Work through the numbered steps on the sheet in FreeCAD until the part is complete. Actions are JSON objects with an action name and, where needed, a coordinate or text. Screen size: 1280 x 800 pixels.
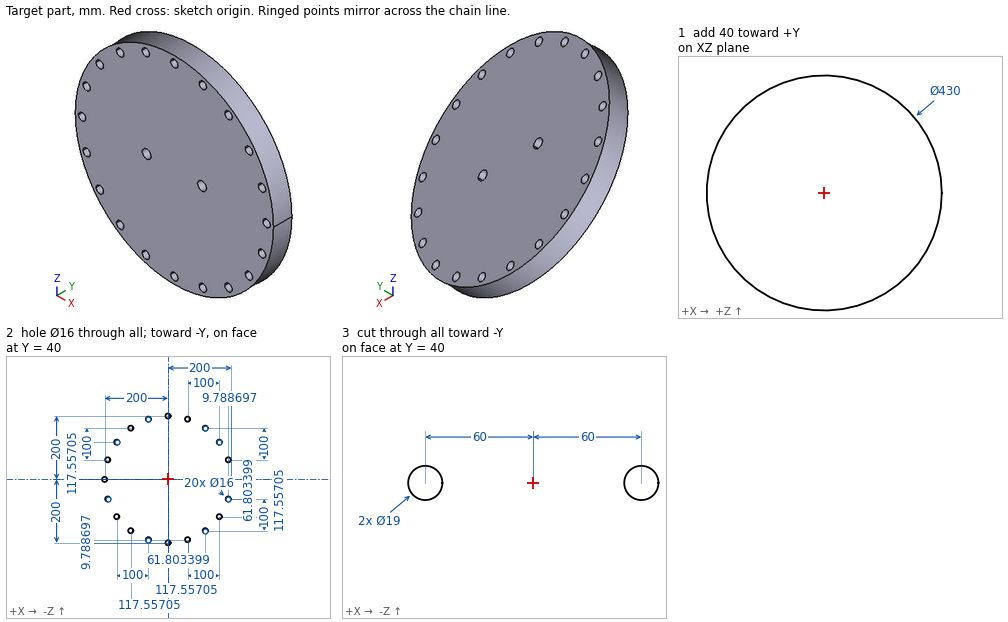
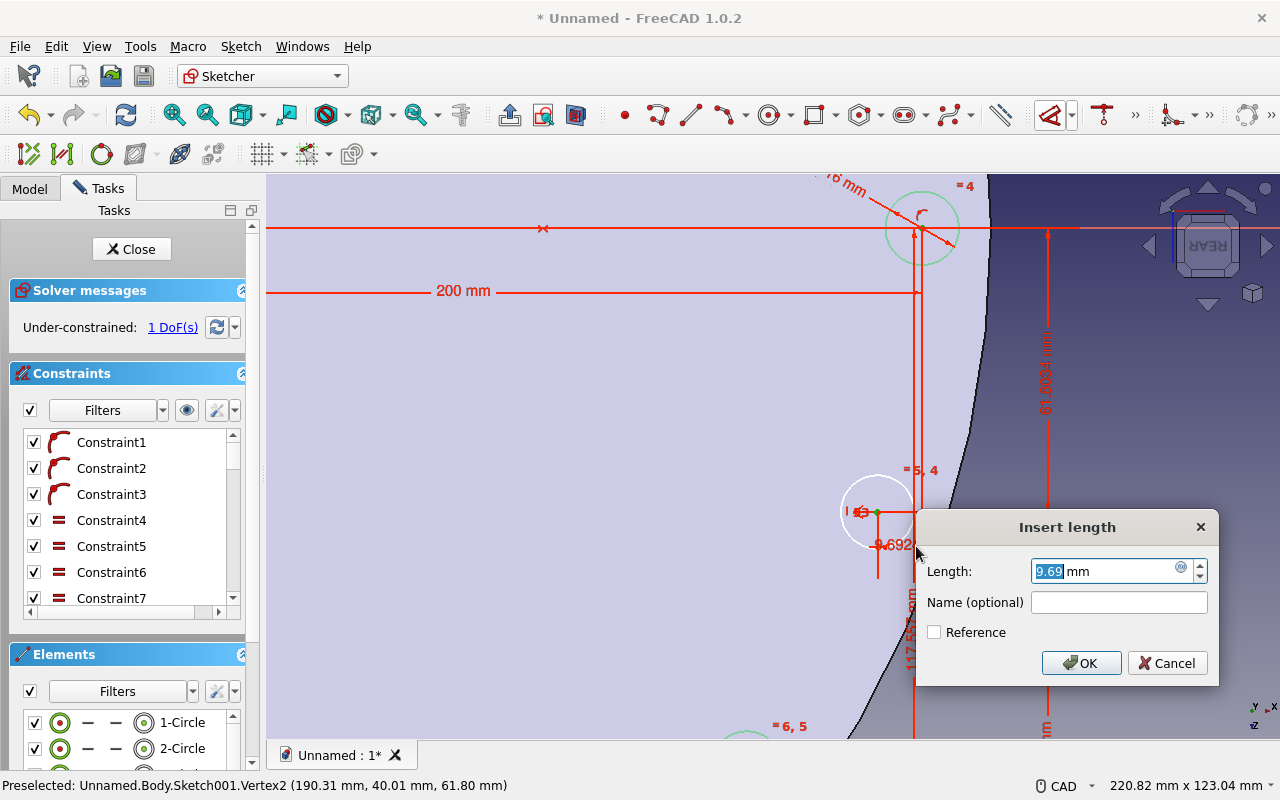
{"action": "type", "text": "9.788697"}
{"action": "key", "text": "Return"}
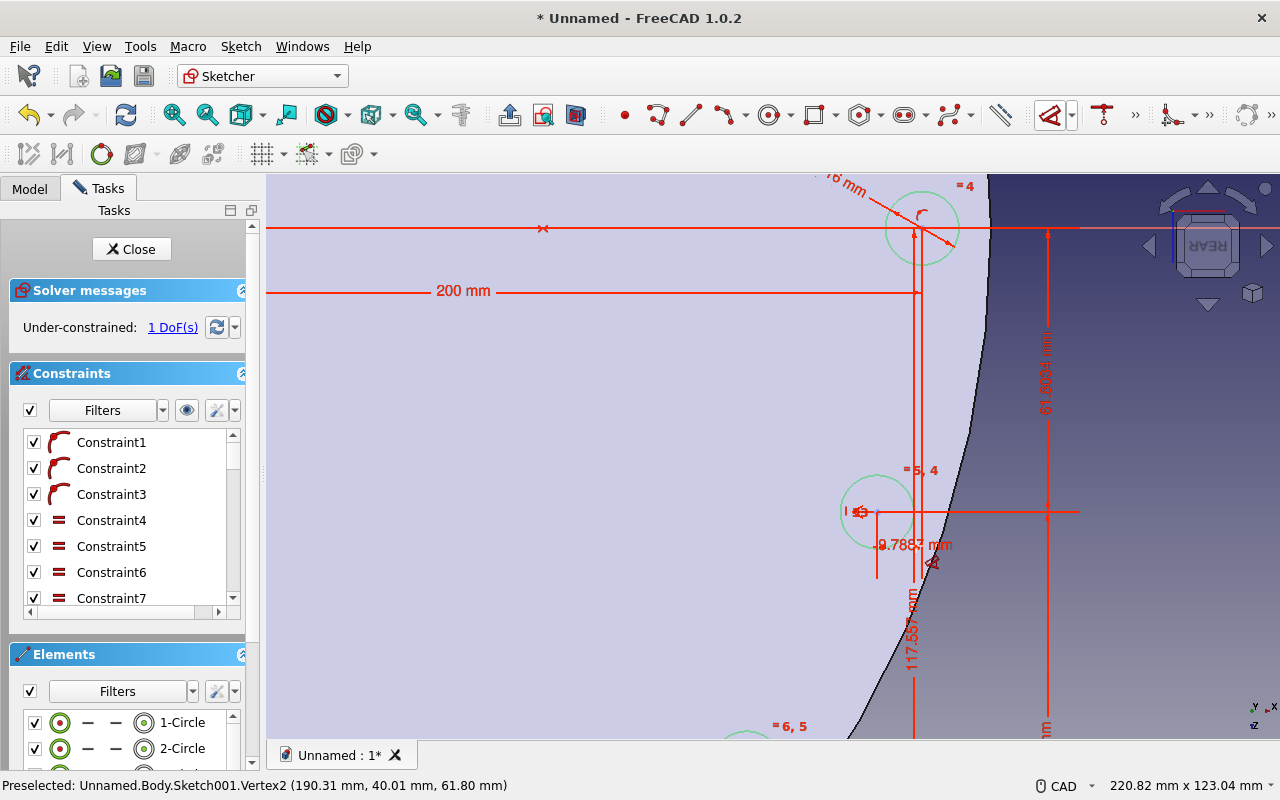
{"action": "scroll", "coordinate": [882, 514], "scroll_direction": "down", "scroll_amount": 8}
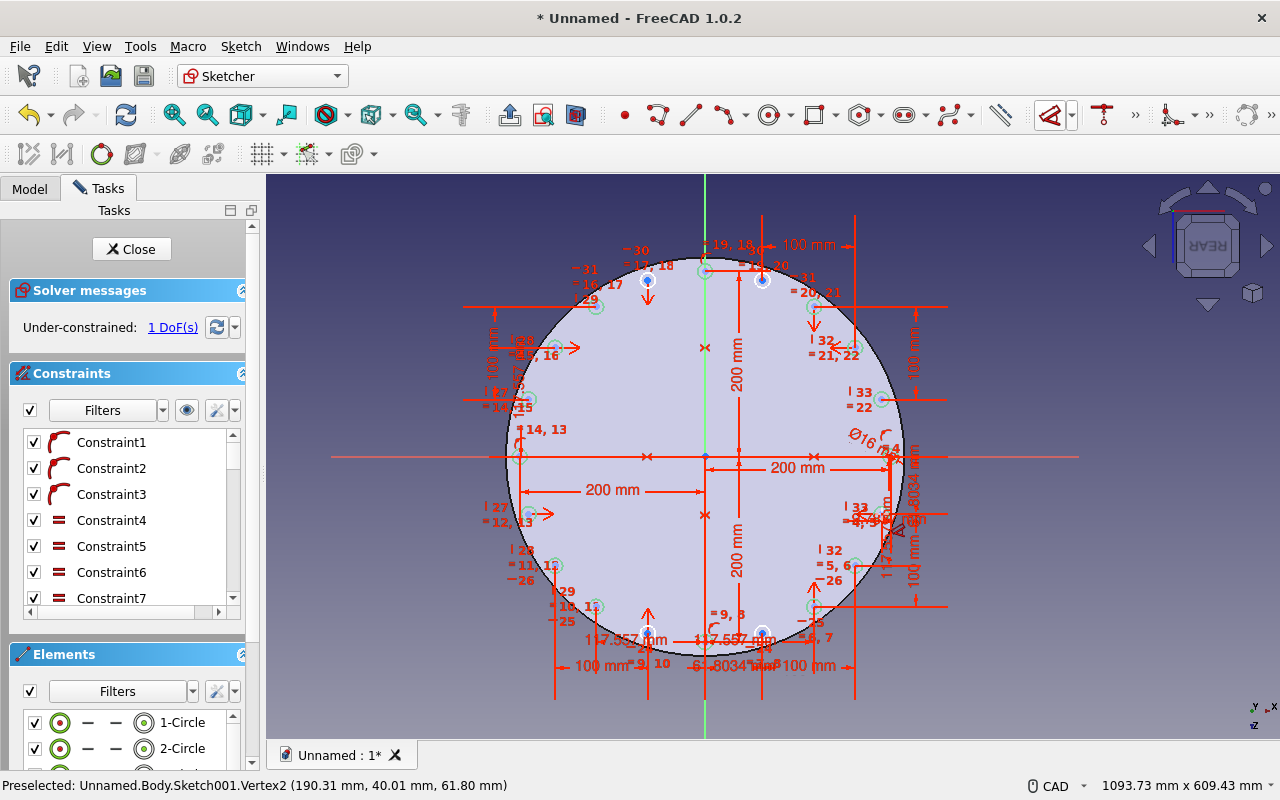
{"action": "scroll", "coordinate": [762, 633], "scroll_direction": "up", "scroll_amount": 8}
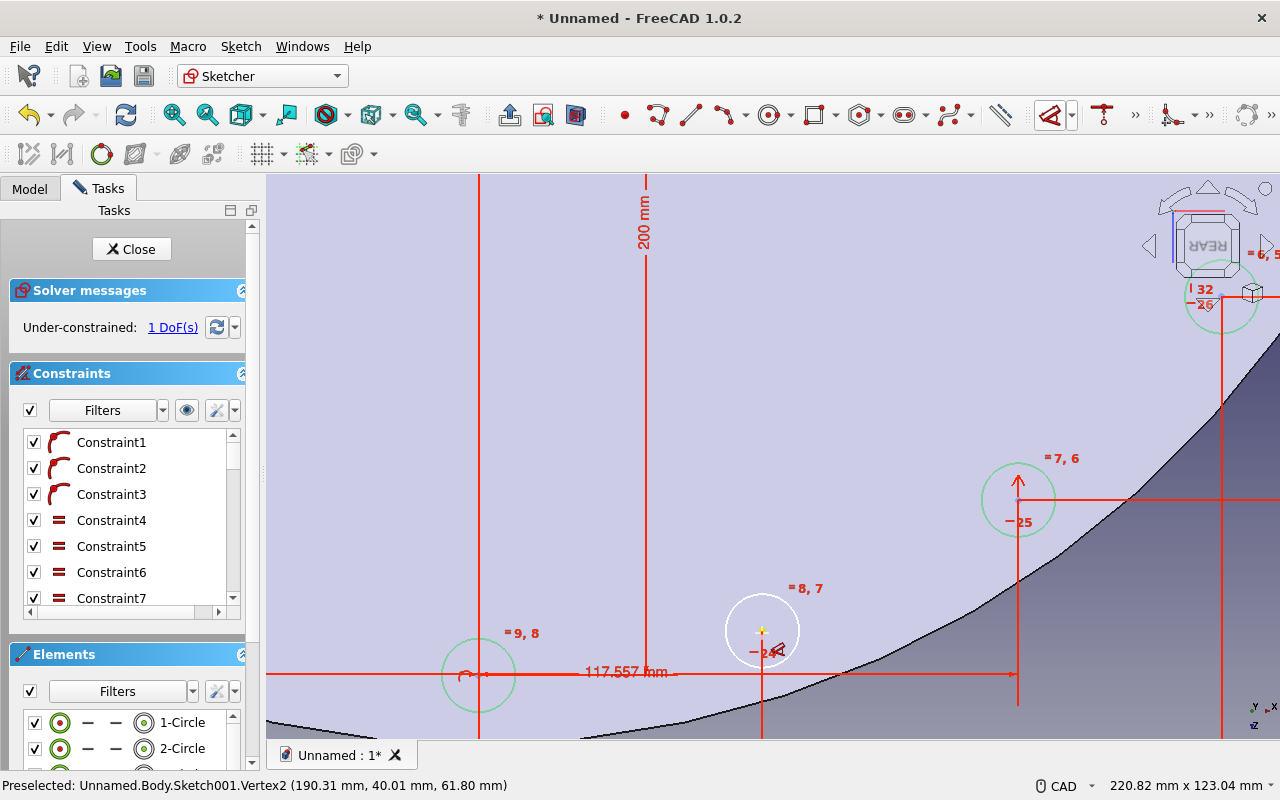
{"action": "left_click", "coordinate": [762, 631]}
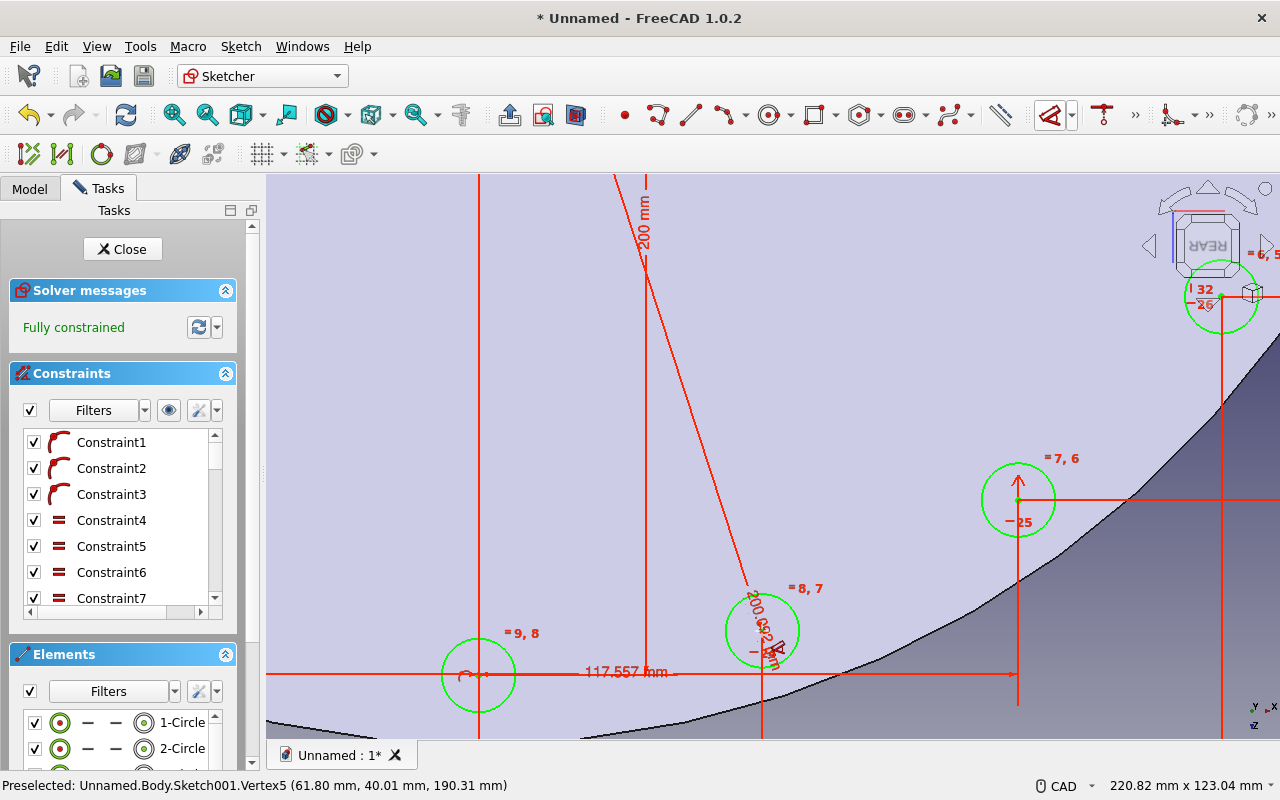
{"action": "left_click", "coordinate": [479, 675]}
{"action": "left_click", "coordinate": [796, 669]}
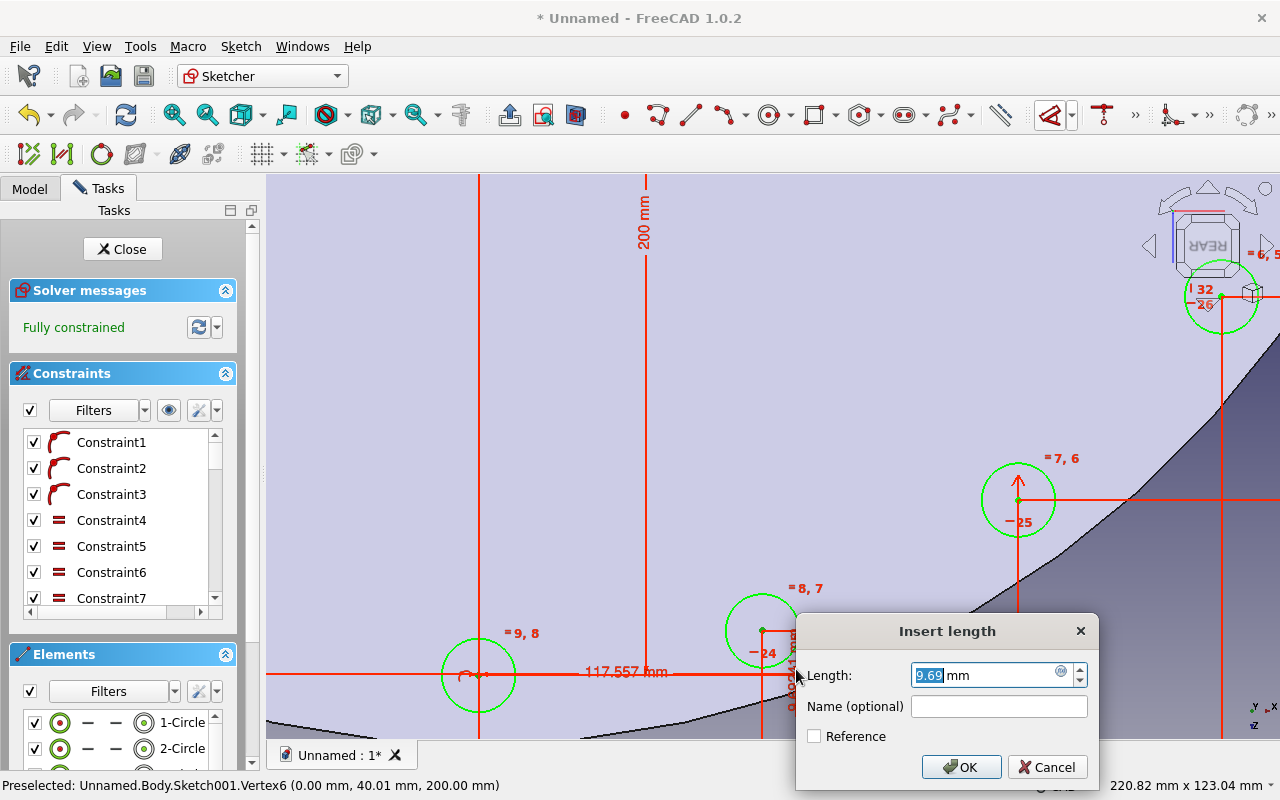
{"action": "type", "text": "9.788697"}
{"action": "key", "text": "Return"}
{"action": "key", "text": "Escape"}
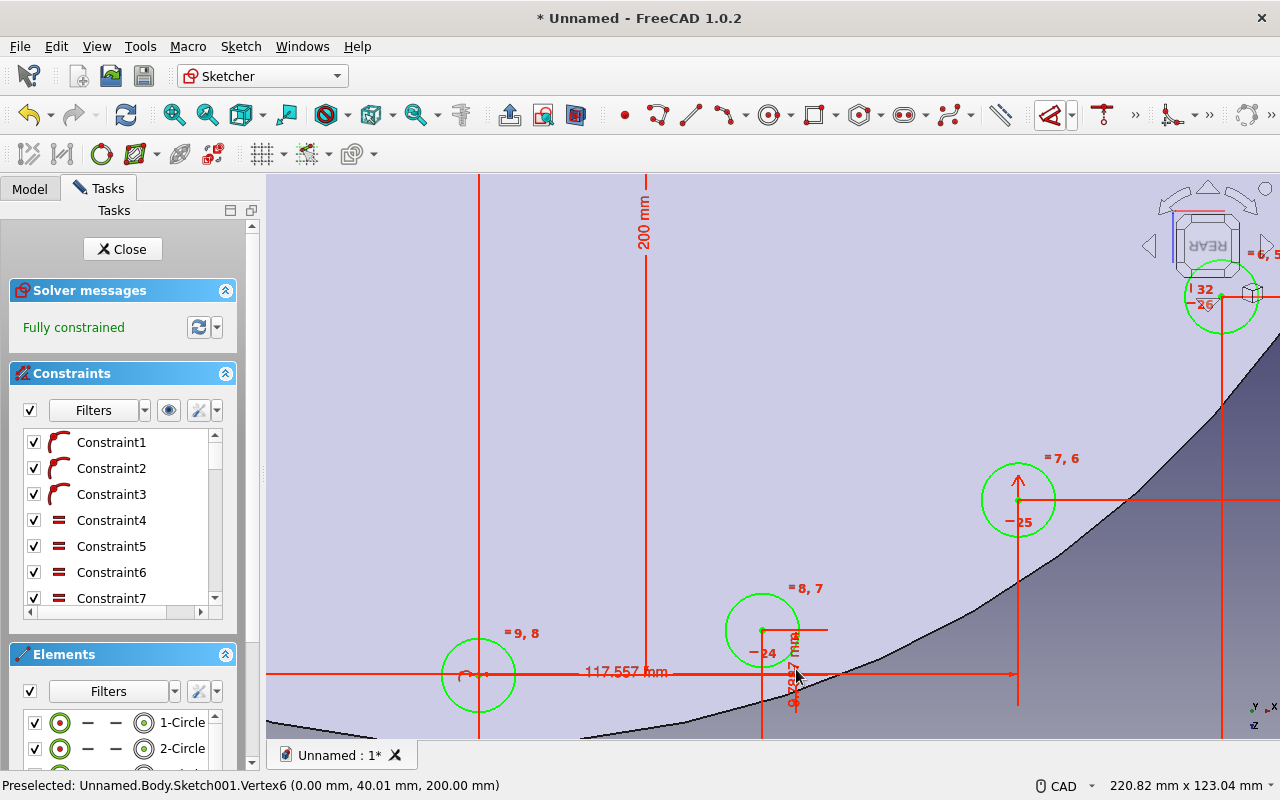
{"action": "left_click", "coordinate": [123, 249]}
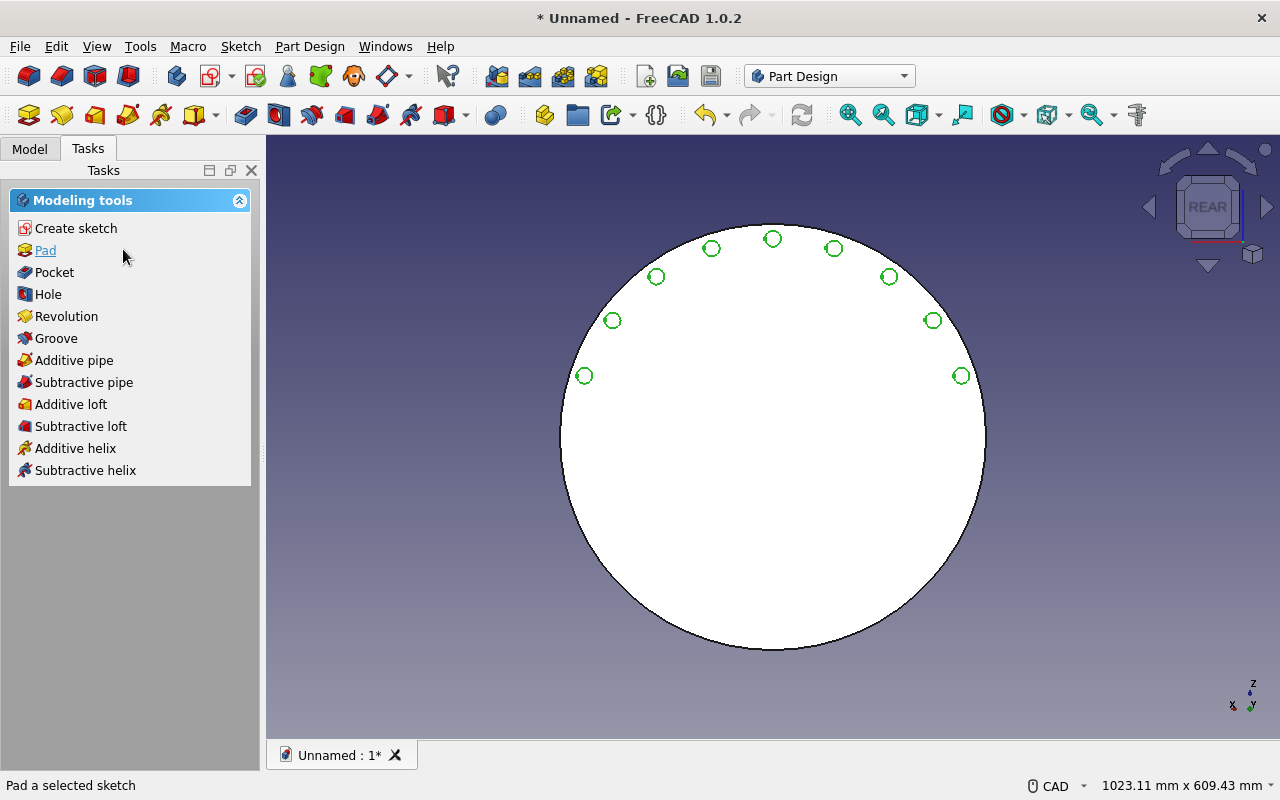
{"action": "left_click", "coordinate": [279, 116]}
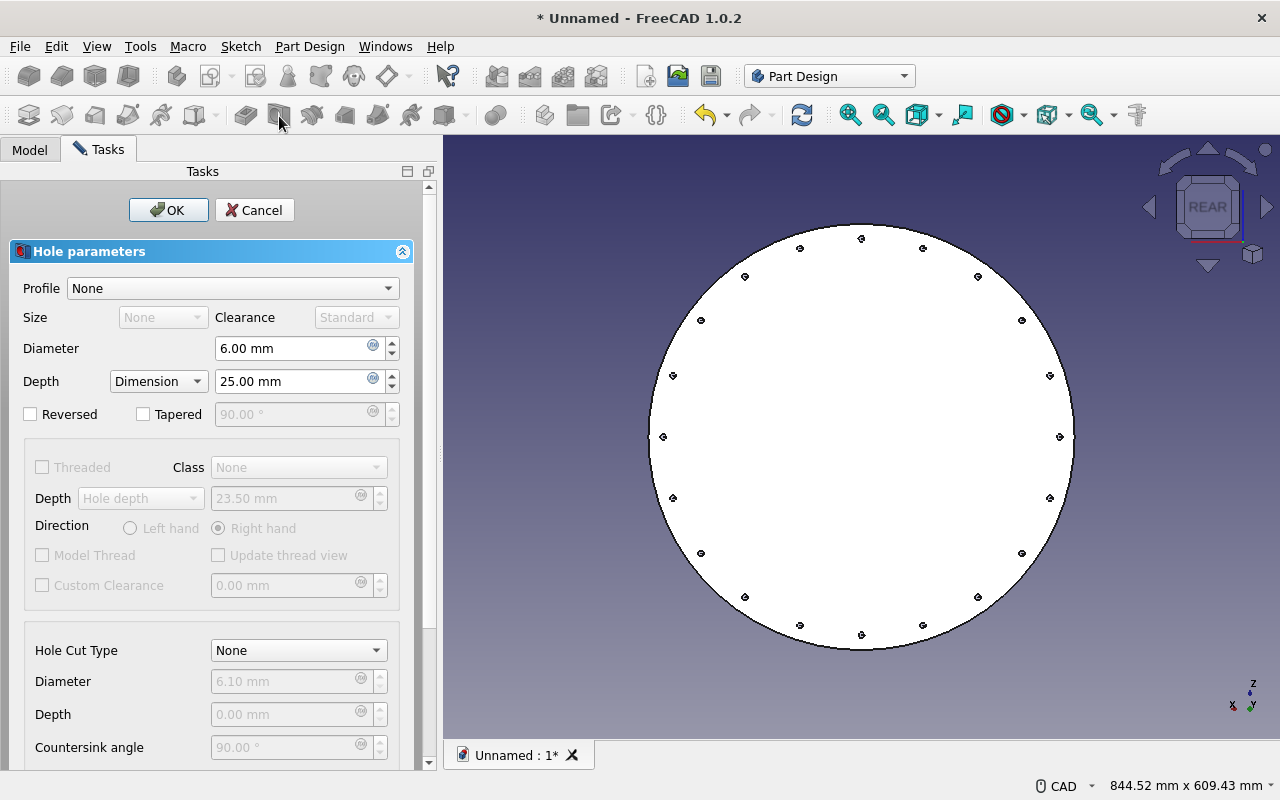
{"action": "triple_click", "coordinate": [300, 348]}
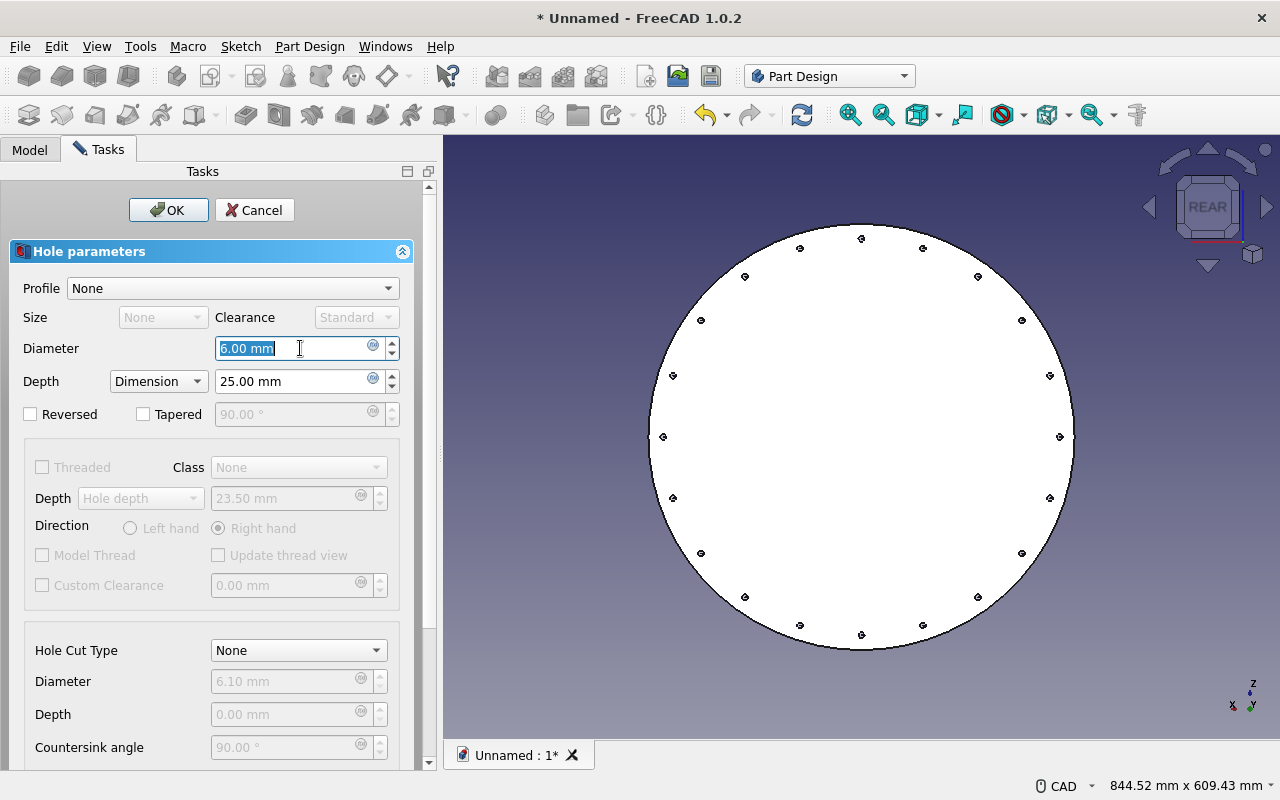
{"action": "type", "text": "16"}
{"action": "key", "text": "Tab"}